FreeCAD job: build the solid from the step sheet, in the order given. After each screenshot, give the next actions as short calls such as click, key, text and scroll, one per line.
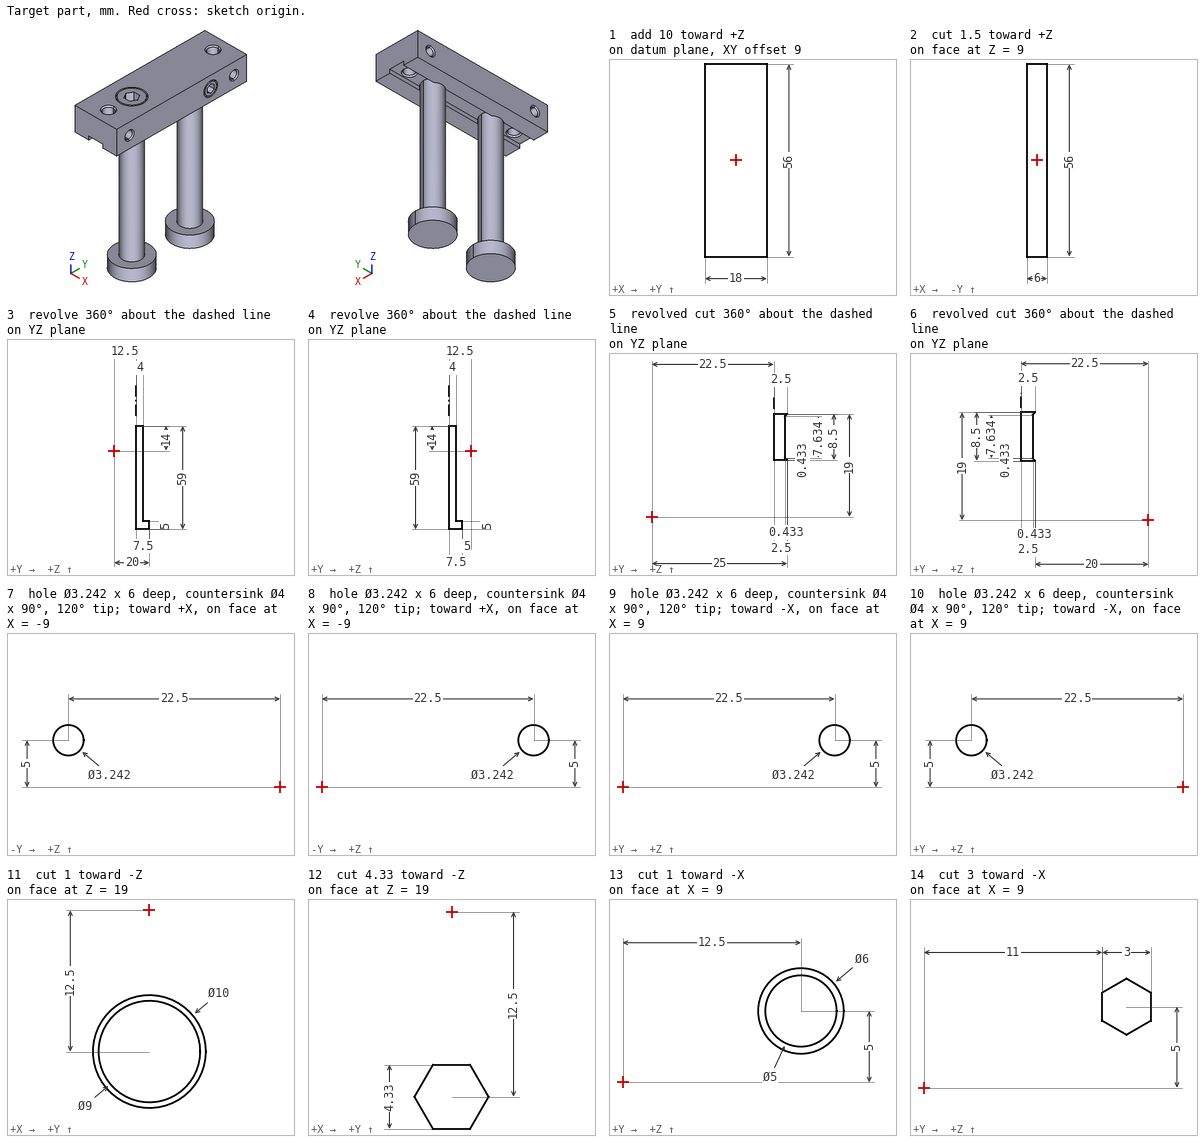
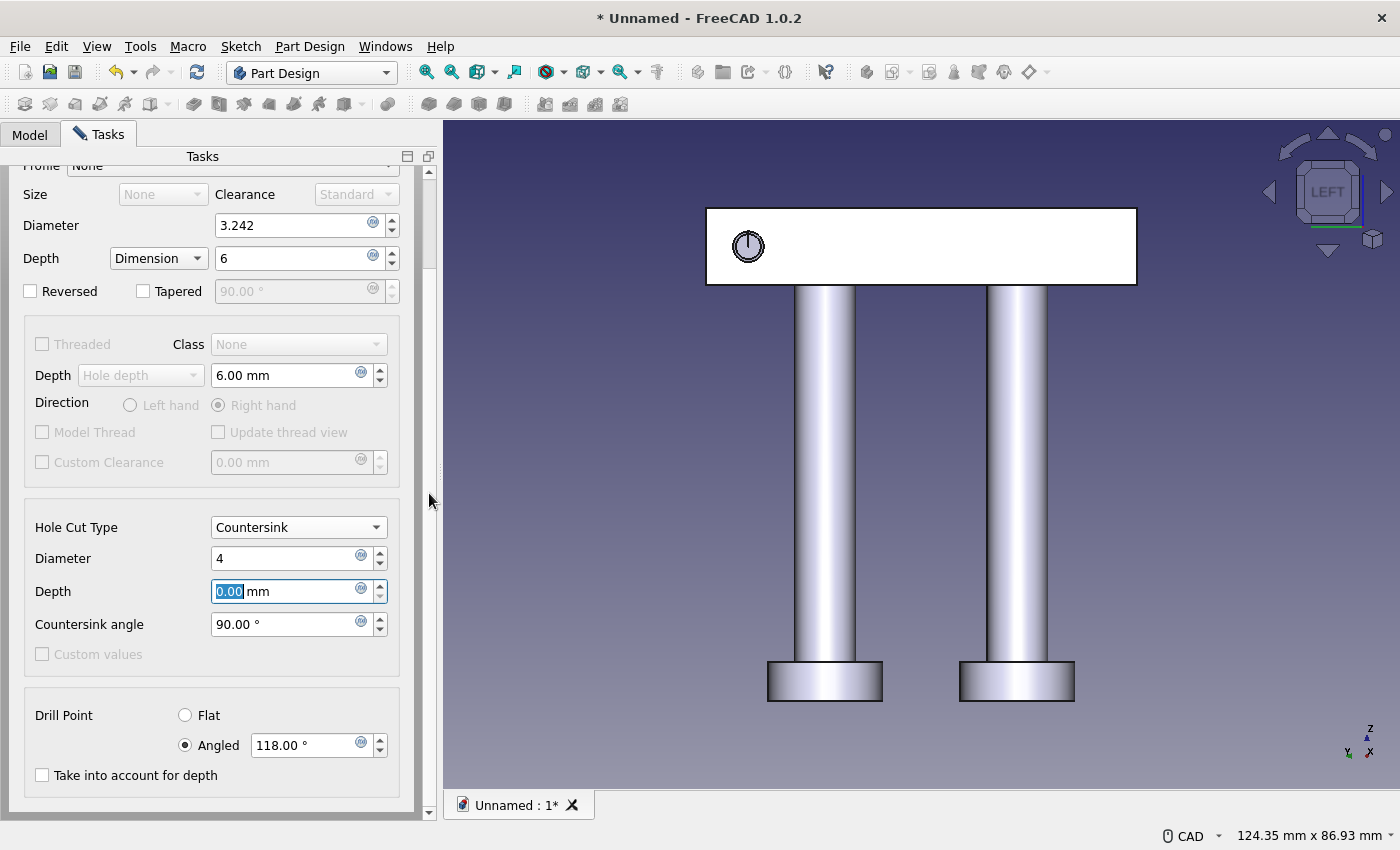
triple_click(312, 746)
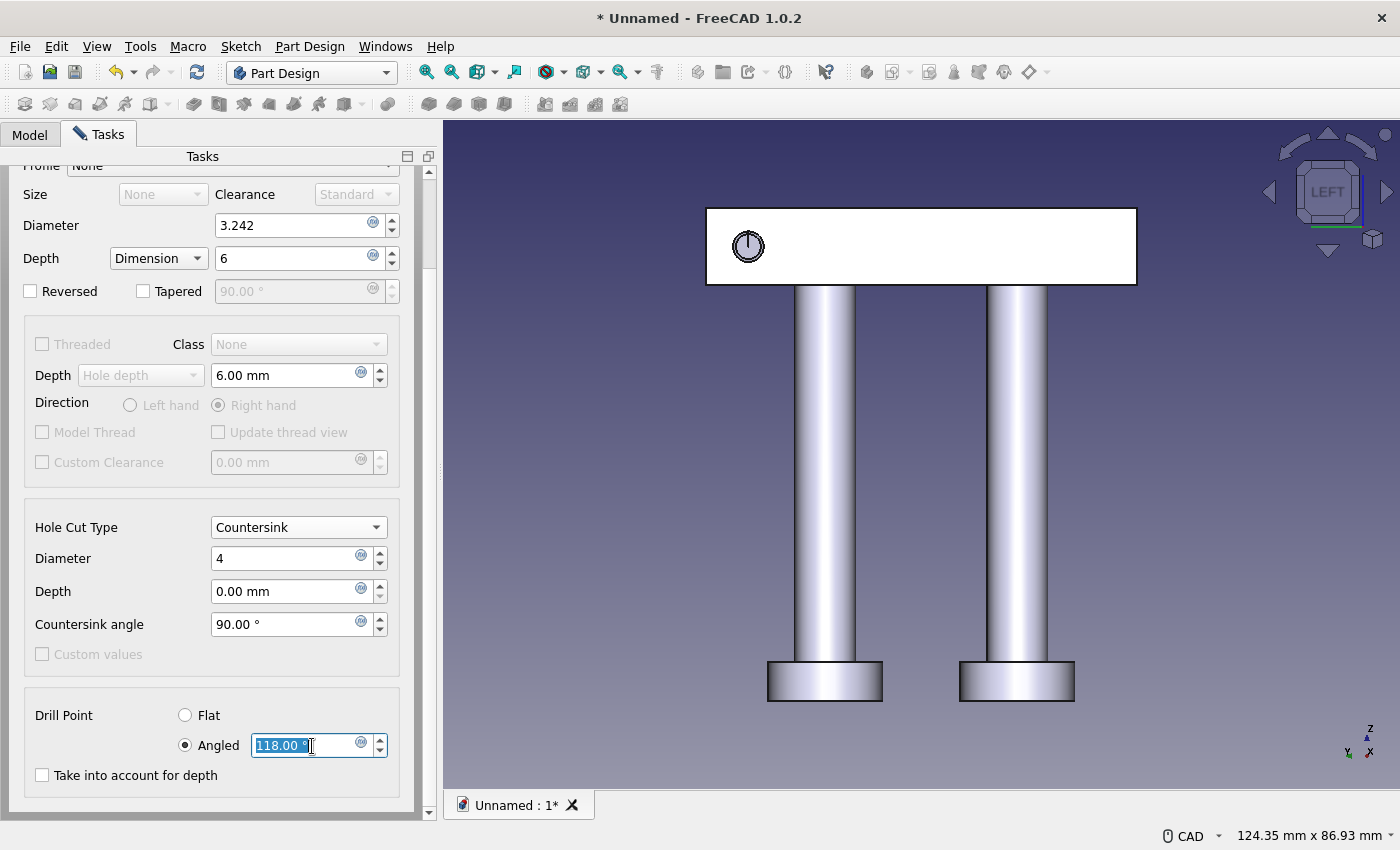
text(120)
key(Tab)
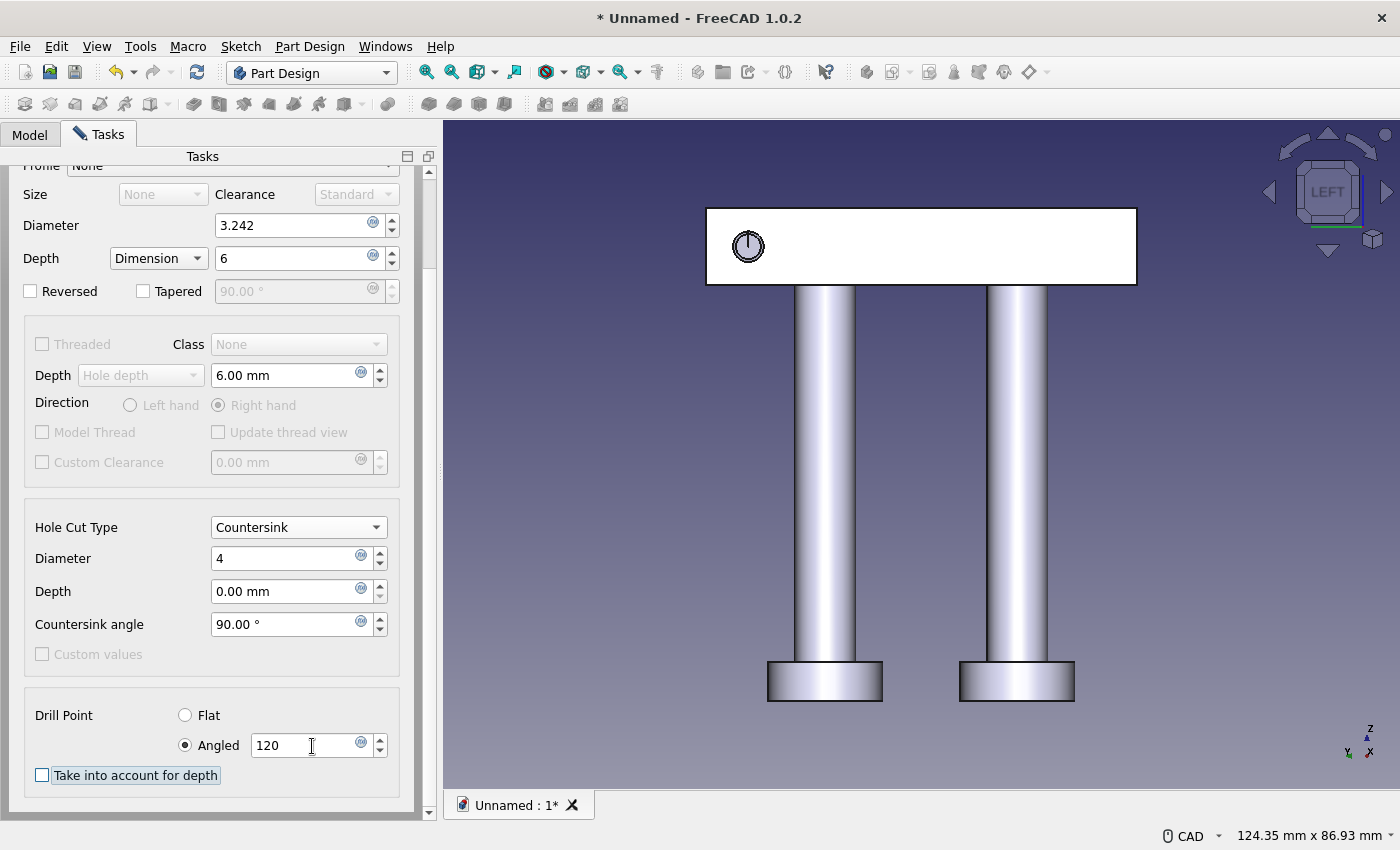
scroll(429, 493, up, 3)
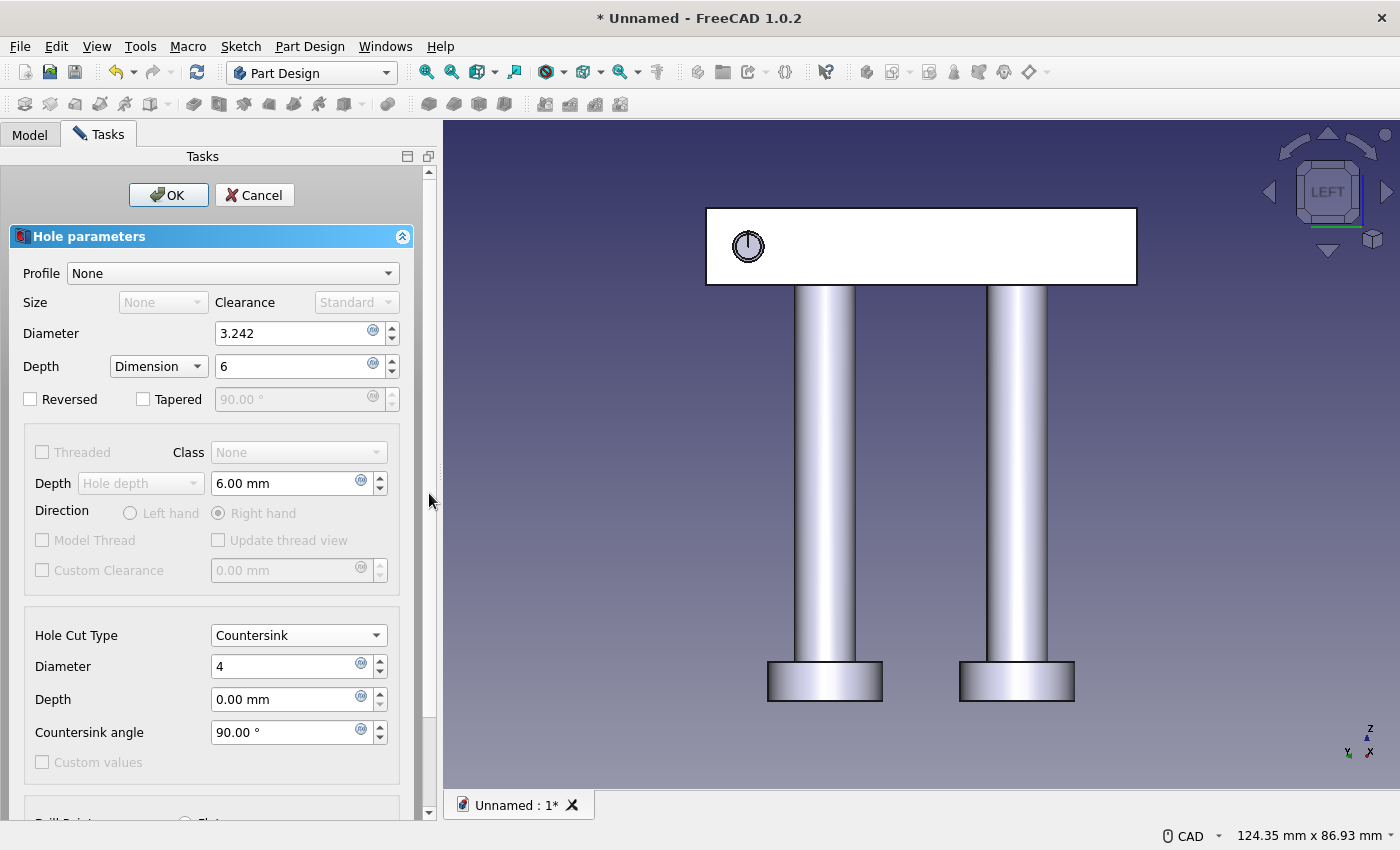
click(169, 195)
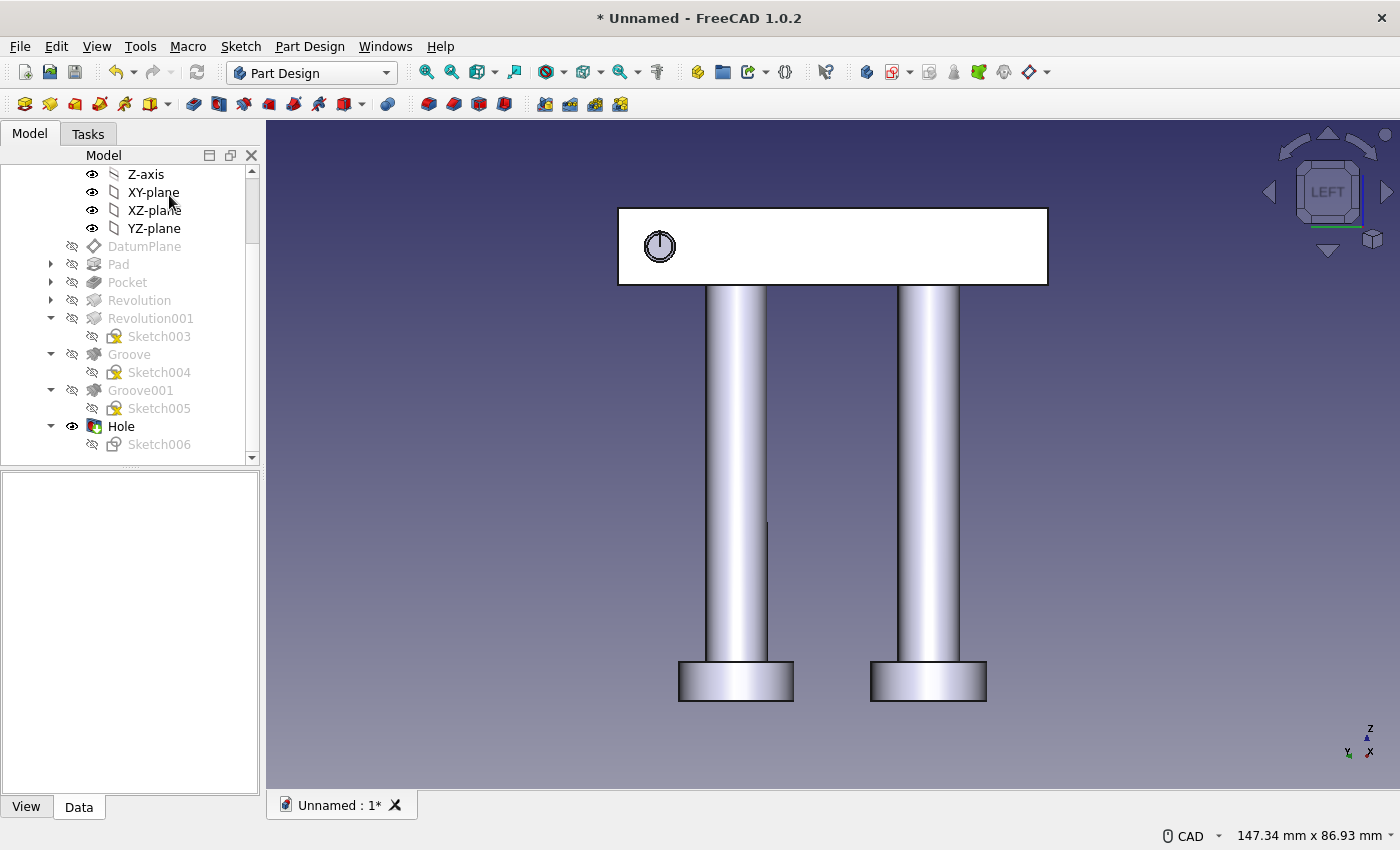
click(771, 246)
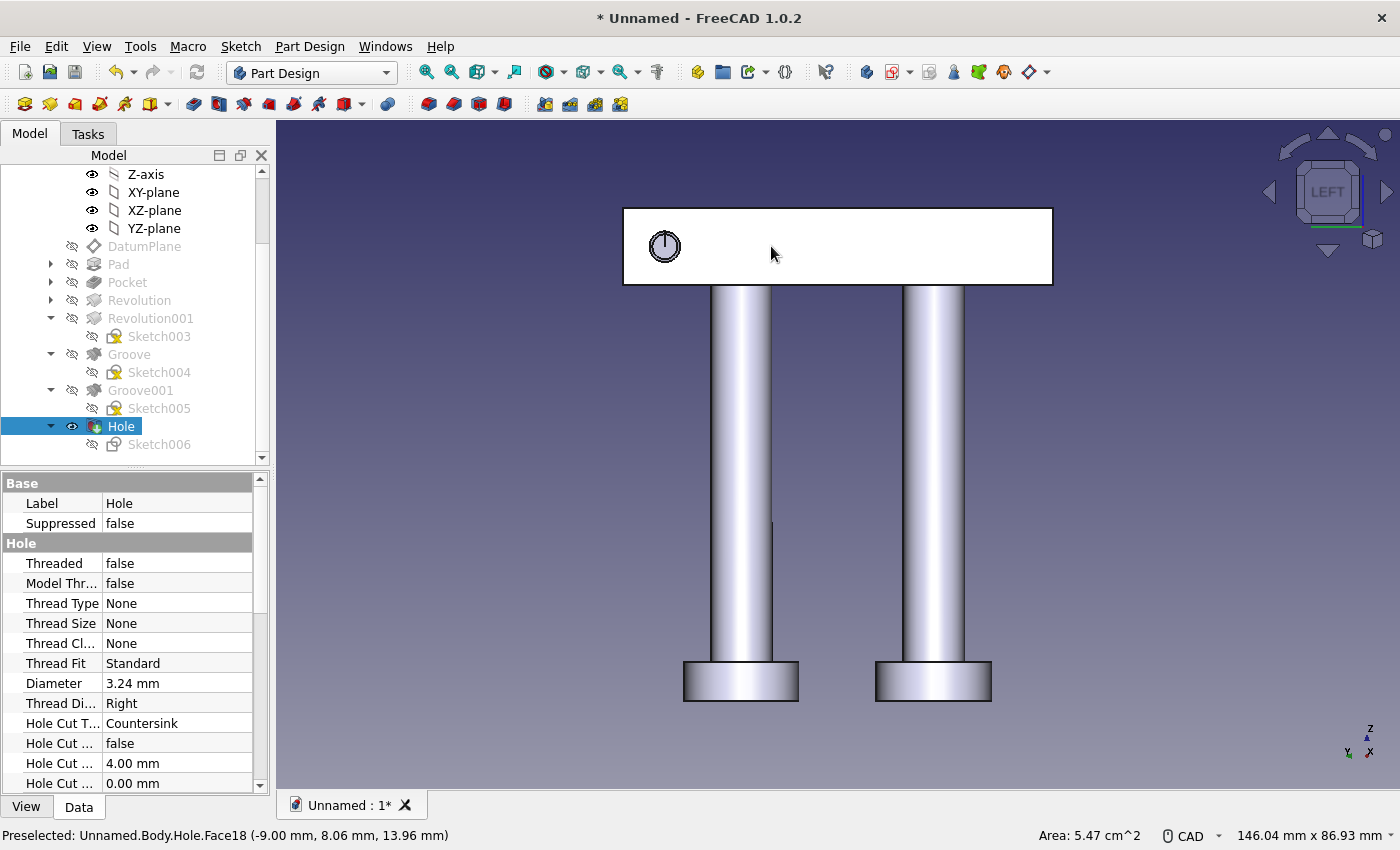
click(892, 72)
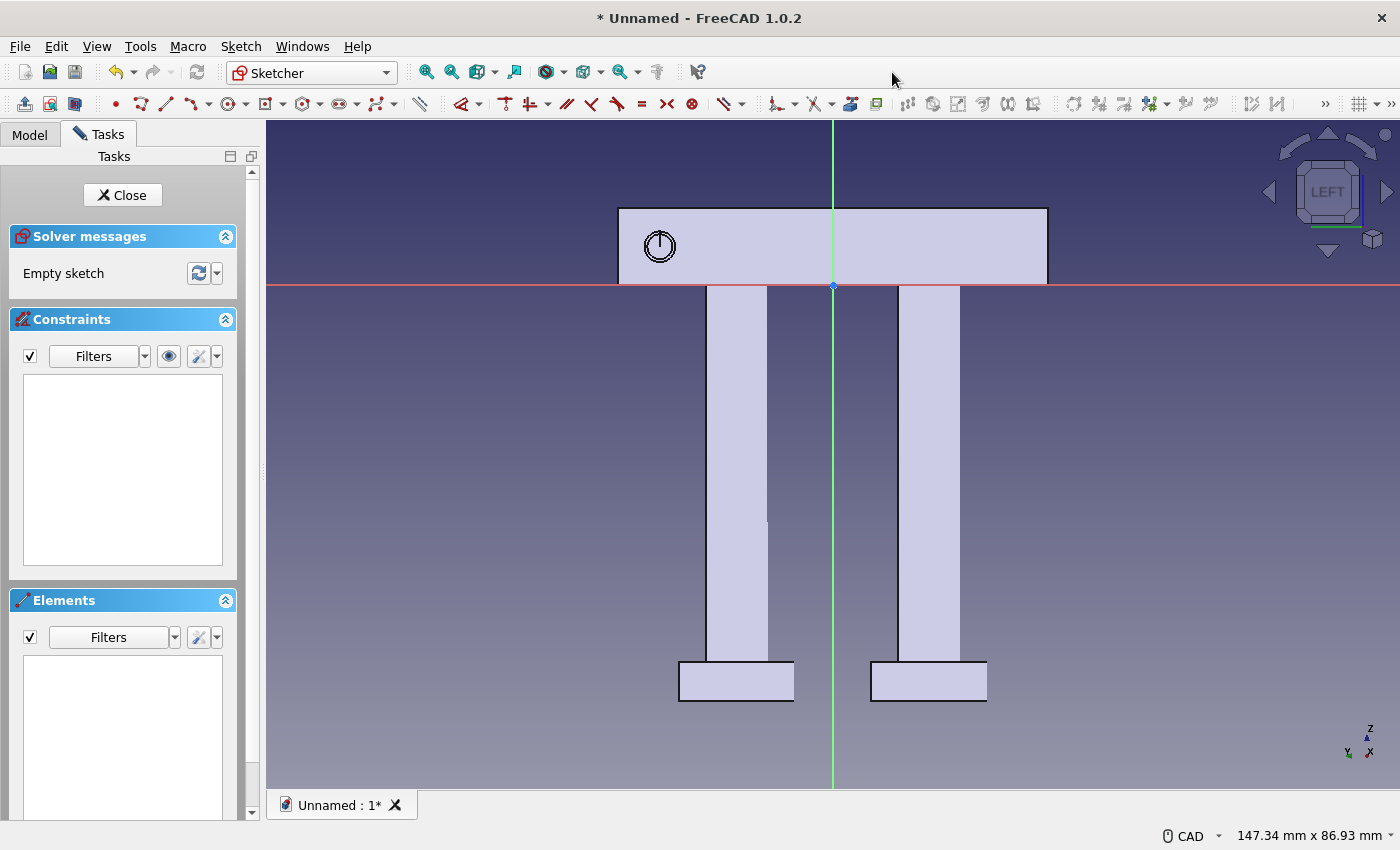
scroll(1022, 233, up, 14)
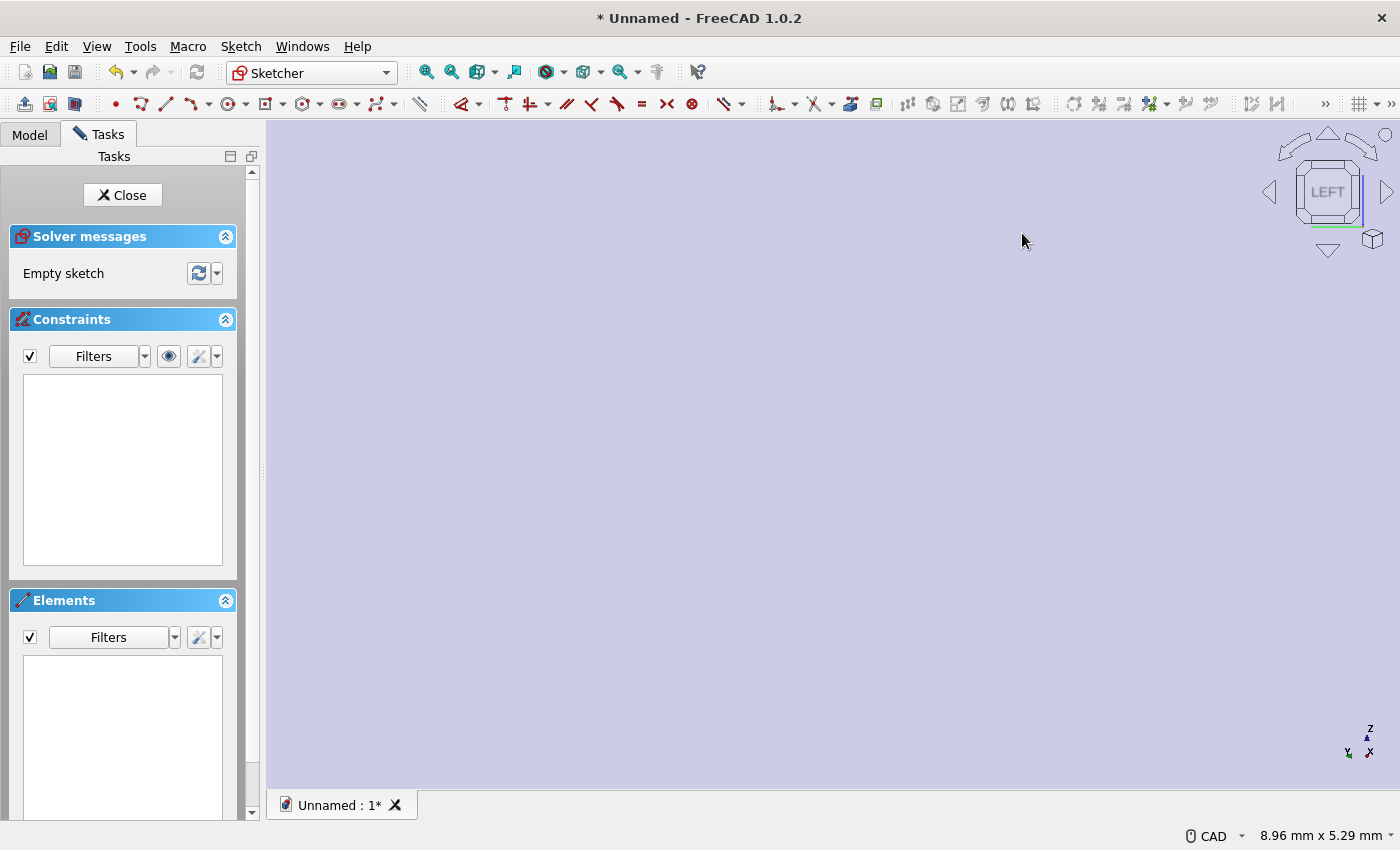
click(228, 104)